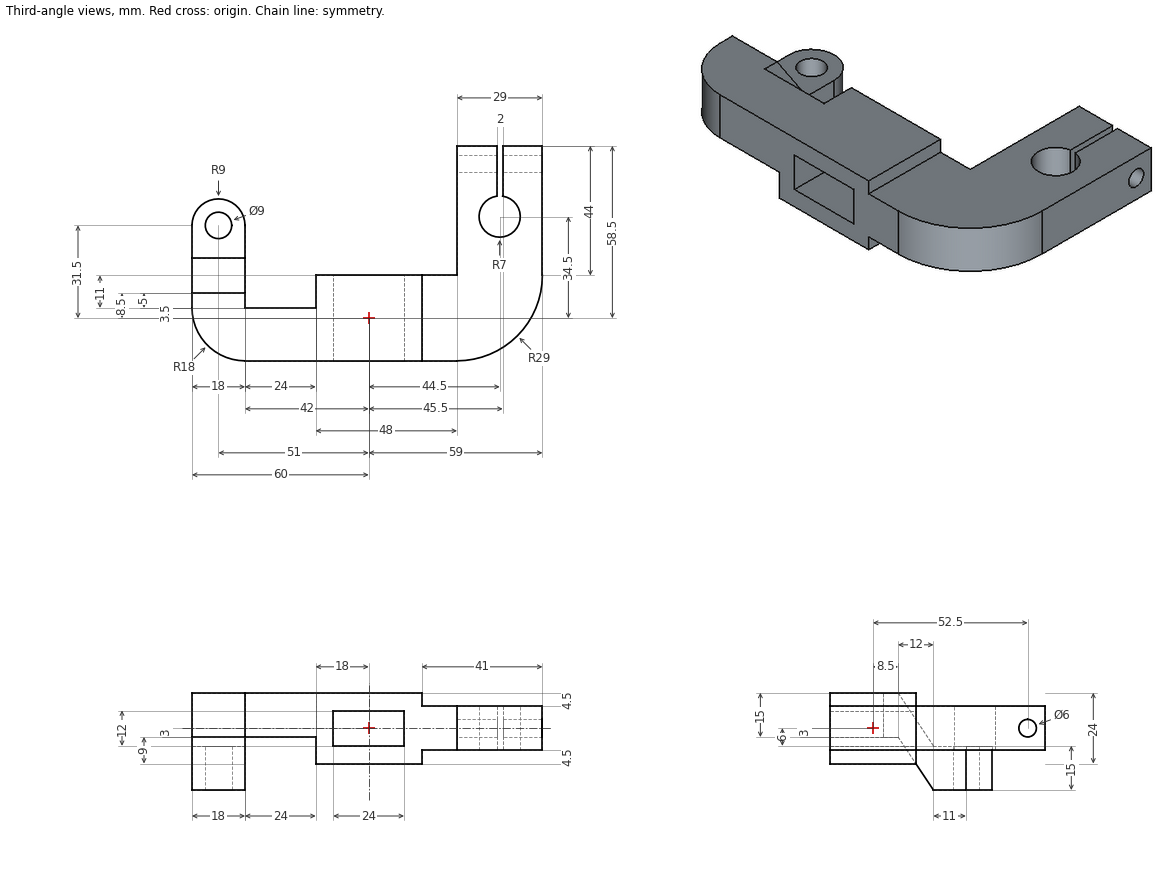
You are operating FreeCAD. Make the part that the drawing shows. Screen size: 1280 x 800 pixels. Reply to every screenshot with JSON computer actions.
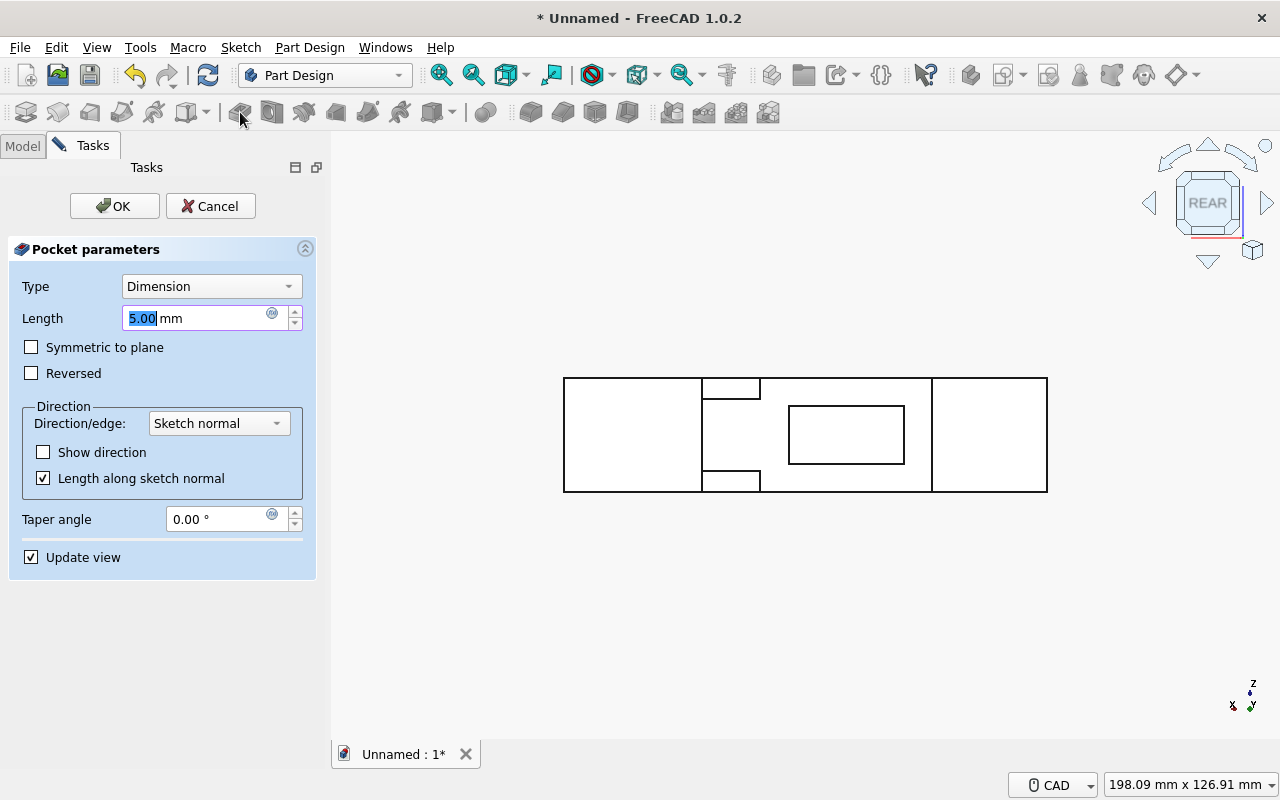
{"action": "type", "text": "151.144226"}
{"action": "key", "text": "Tab"}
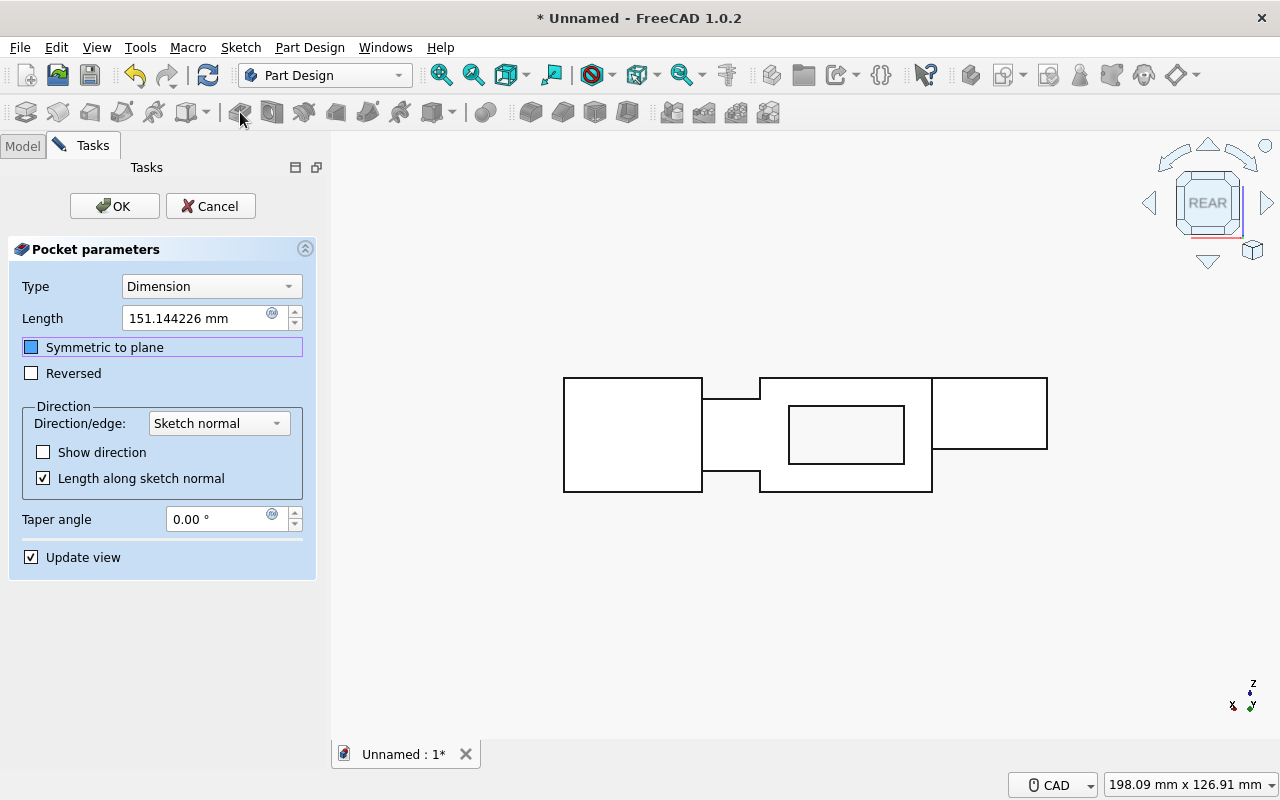
{"action": "left_click", "coordinate": [30, 347]}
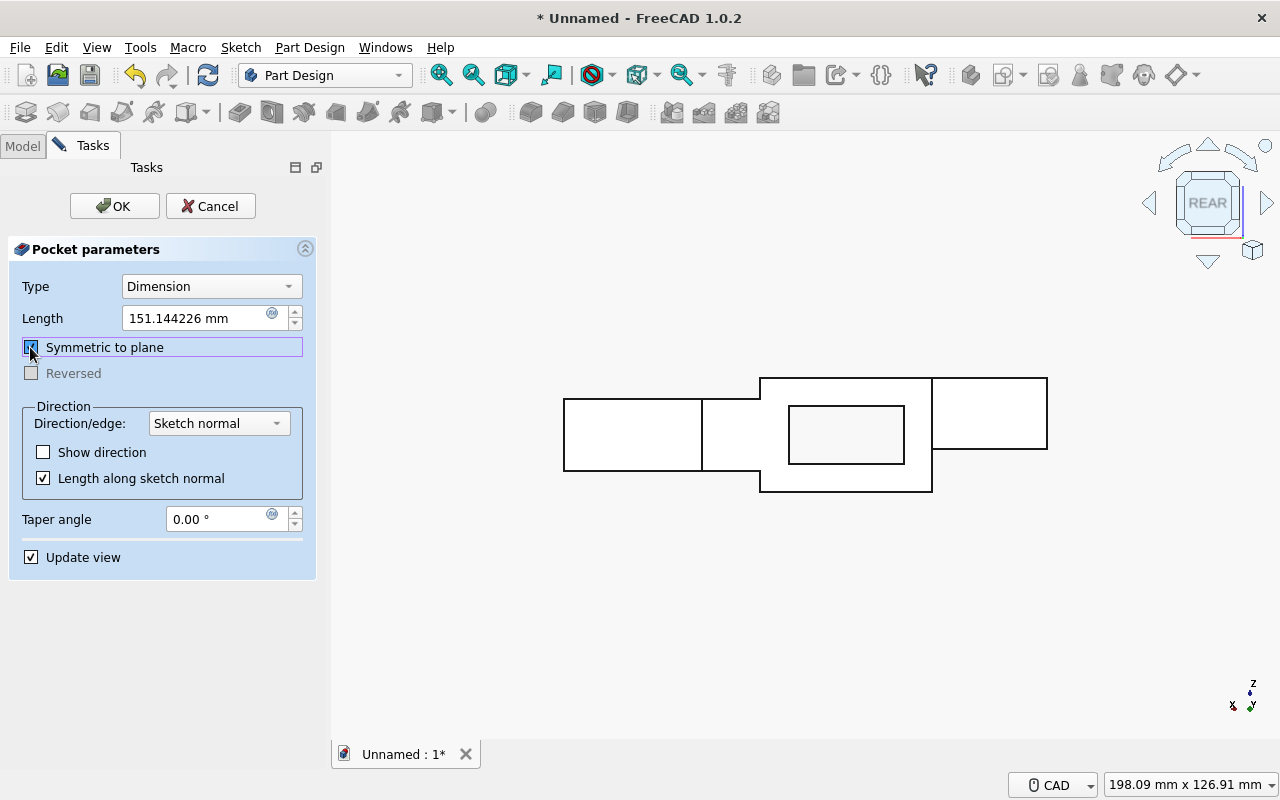
{"action": "left_click", "coordinate": [115, 206]}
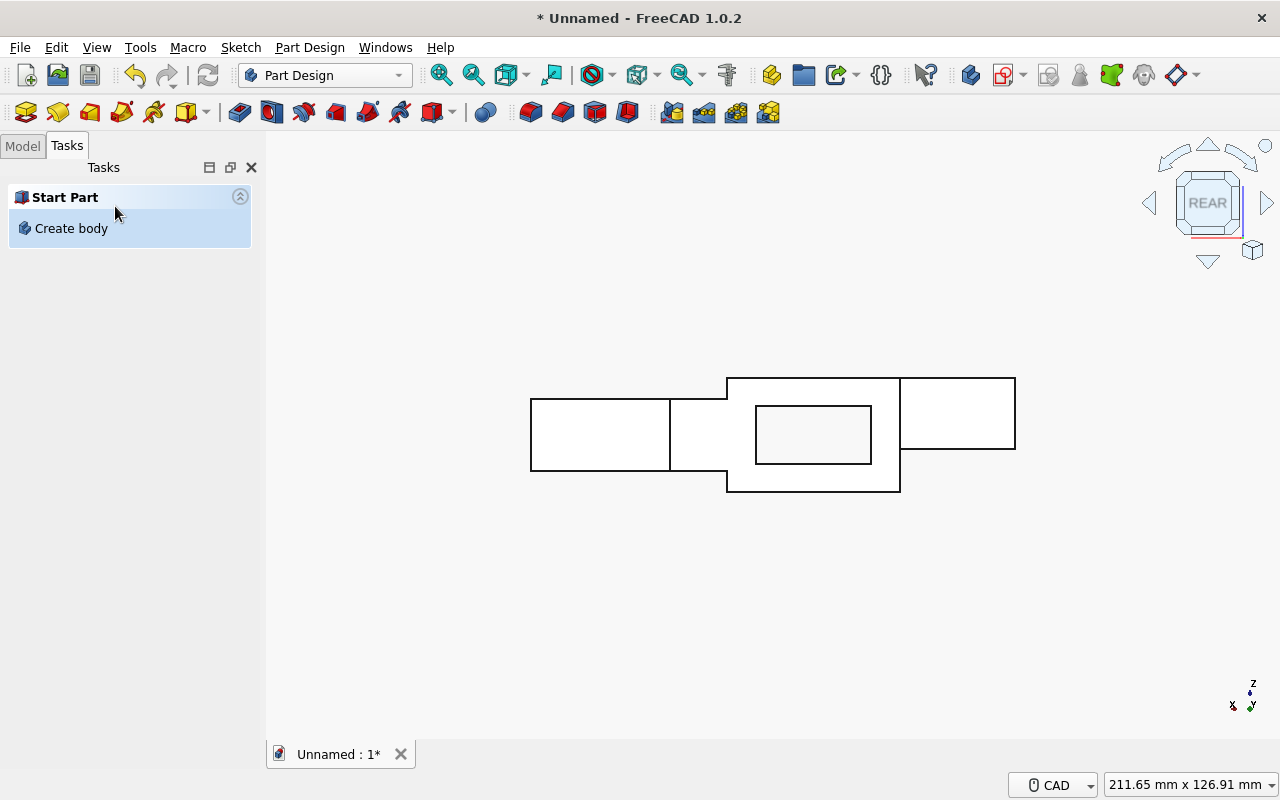
{"action": "key", "text": "0"}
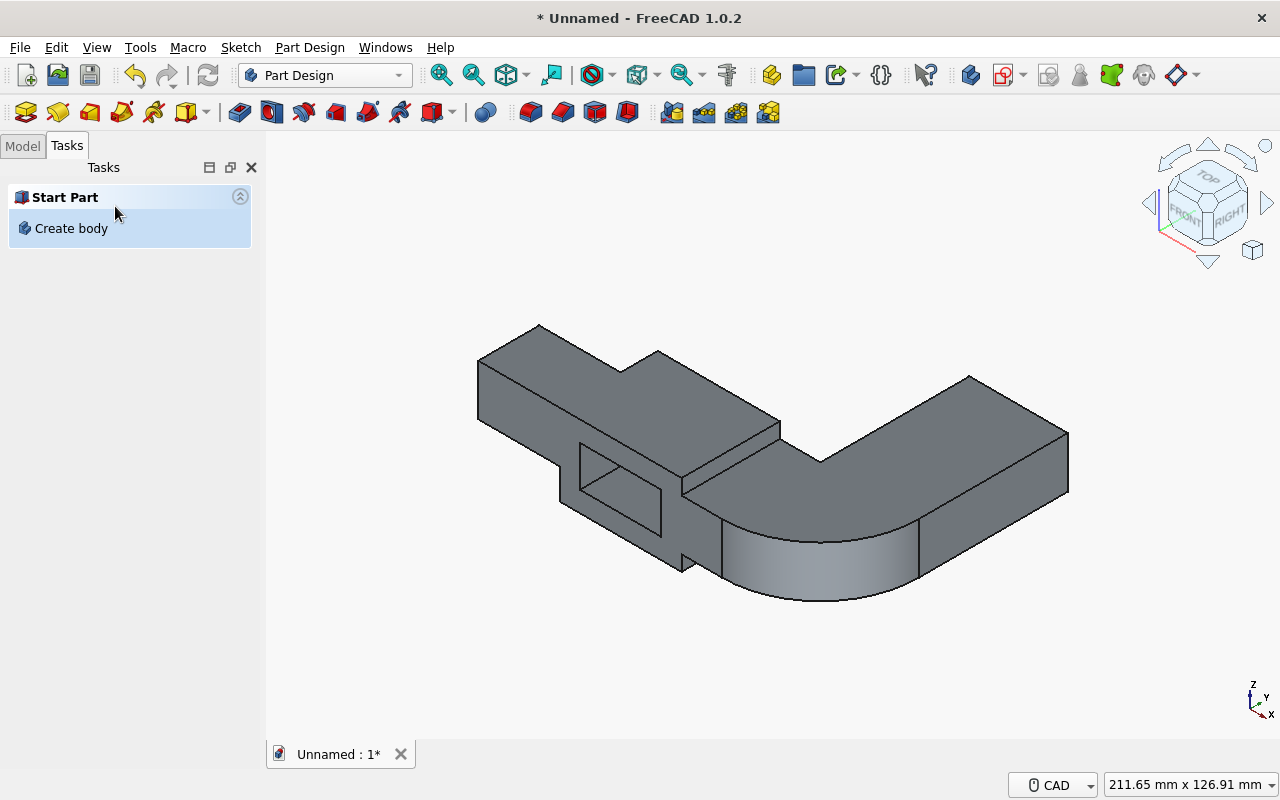
{"action": "left_click", "coordinate": [965, 434]}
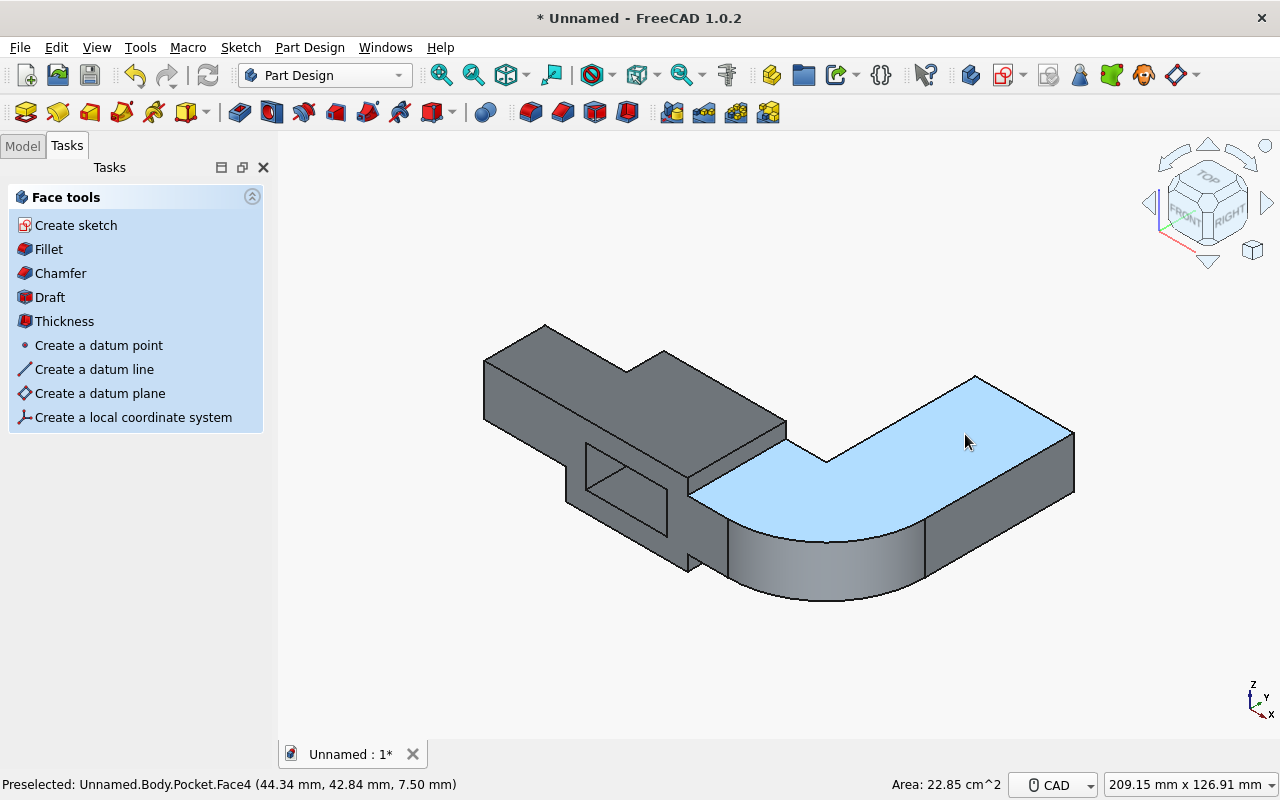
{"action": "left_click", "coordinate": [1004, 76]}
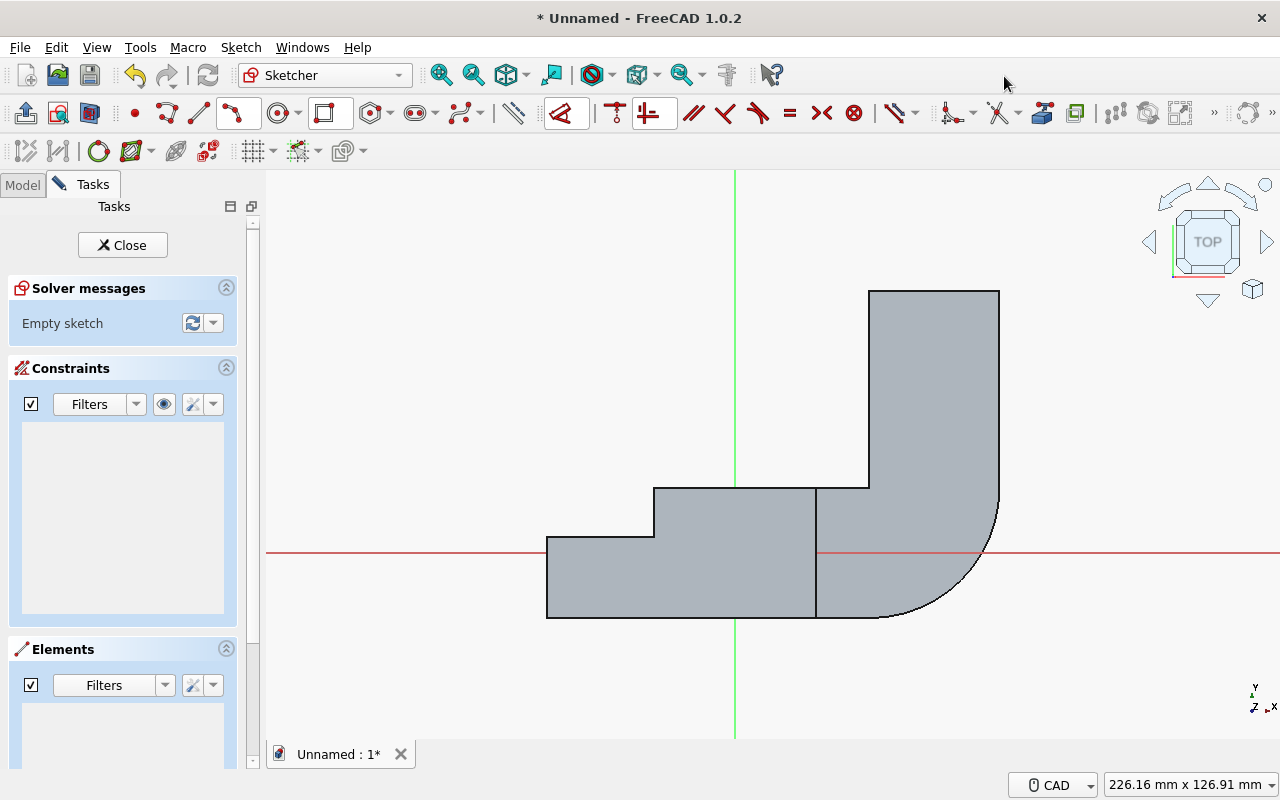
{"action": "scroll", "coordinate": [1106, 356], "scroll_direction": "up", "scroll_amount": 2}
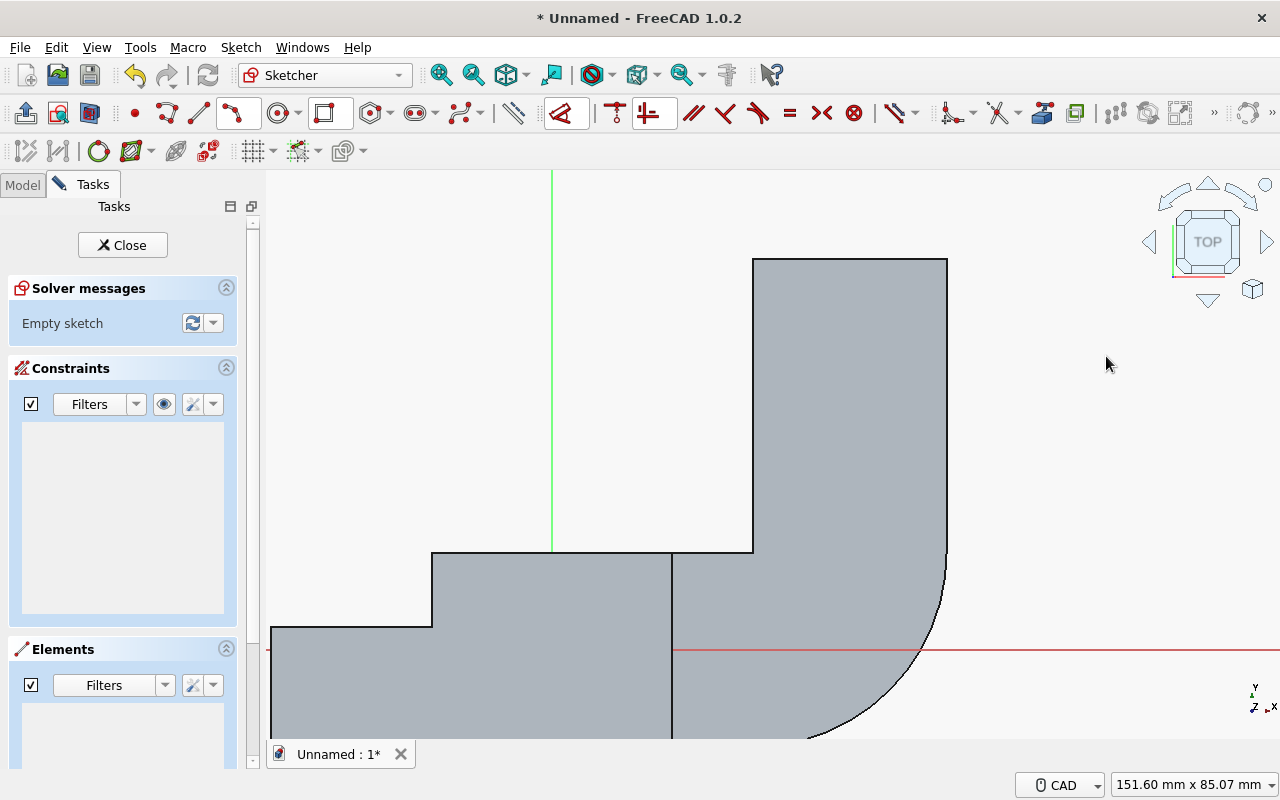
{"action": "left_click", "coordinate": [168, 114]}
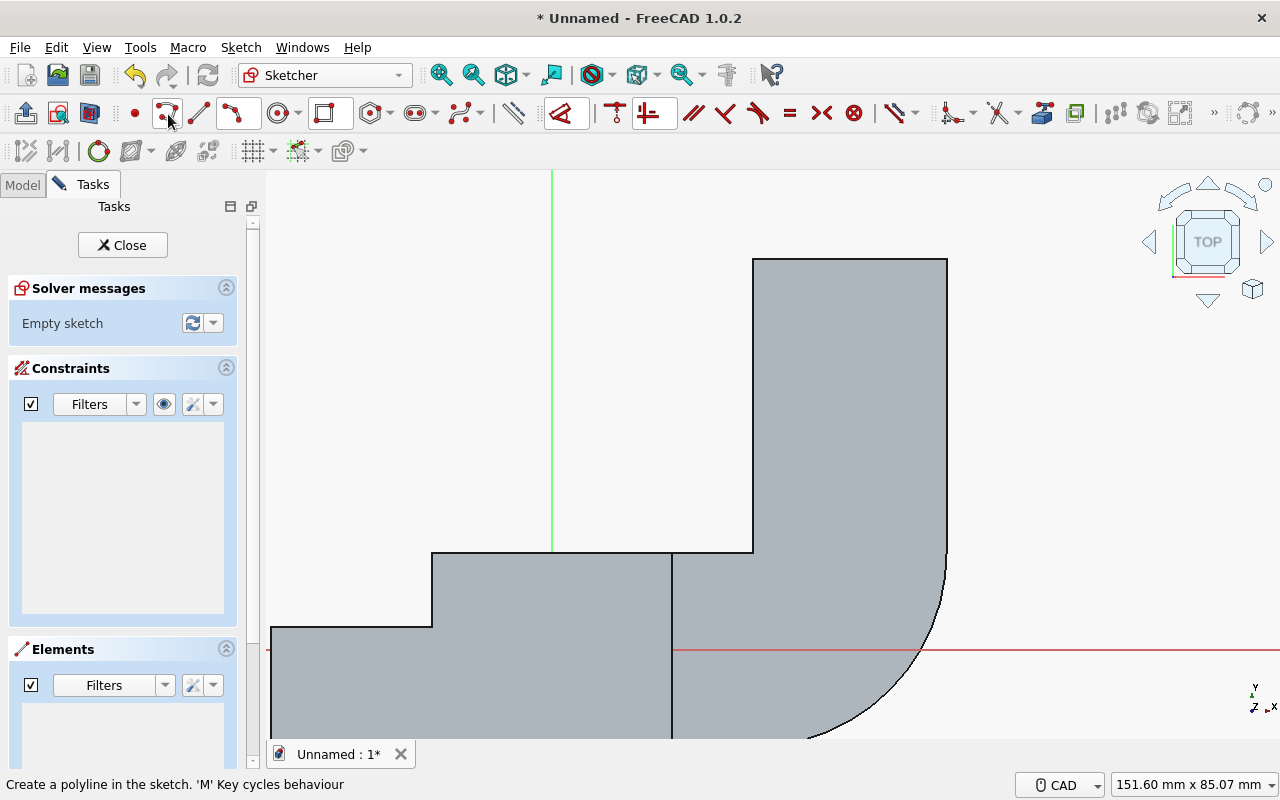
{"action": "left_click", "coordinate": [856, 373]}
{"action": "left_click", "coordinate": [856, 259]}
{"action": "left_click", "coordinate": [843, 259]}
{"action": "left_click", "coordinate": [843, 373]}
{"action": "right_click", "coordinate": [843, 373]}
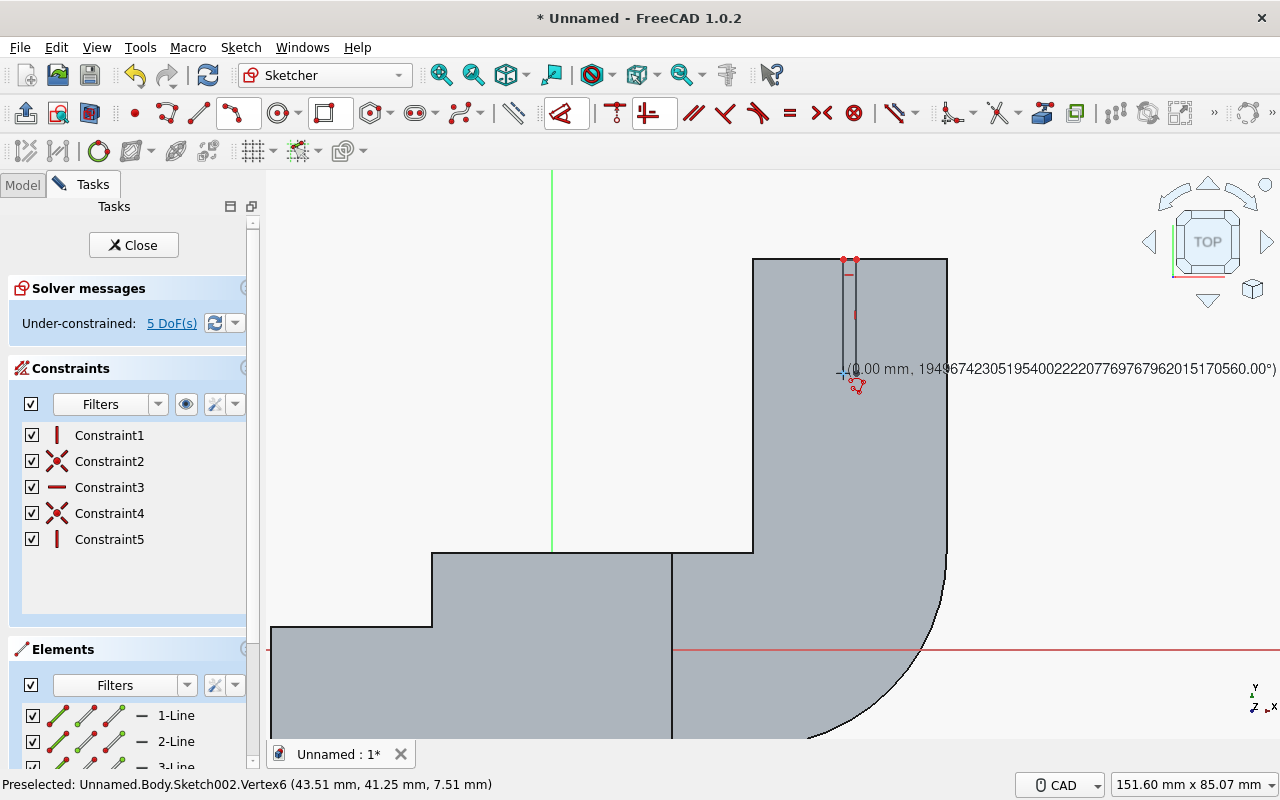
{"action": "left_click", "coordinate": [232, 114]}